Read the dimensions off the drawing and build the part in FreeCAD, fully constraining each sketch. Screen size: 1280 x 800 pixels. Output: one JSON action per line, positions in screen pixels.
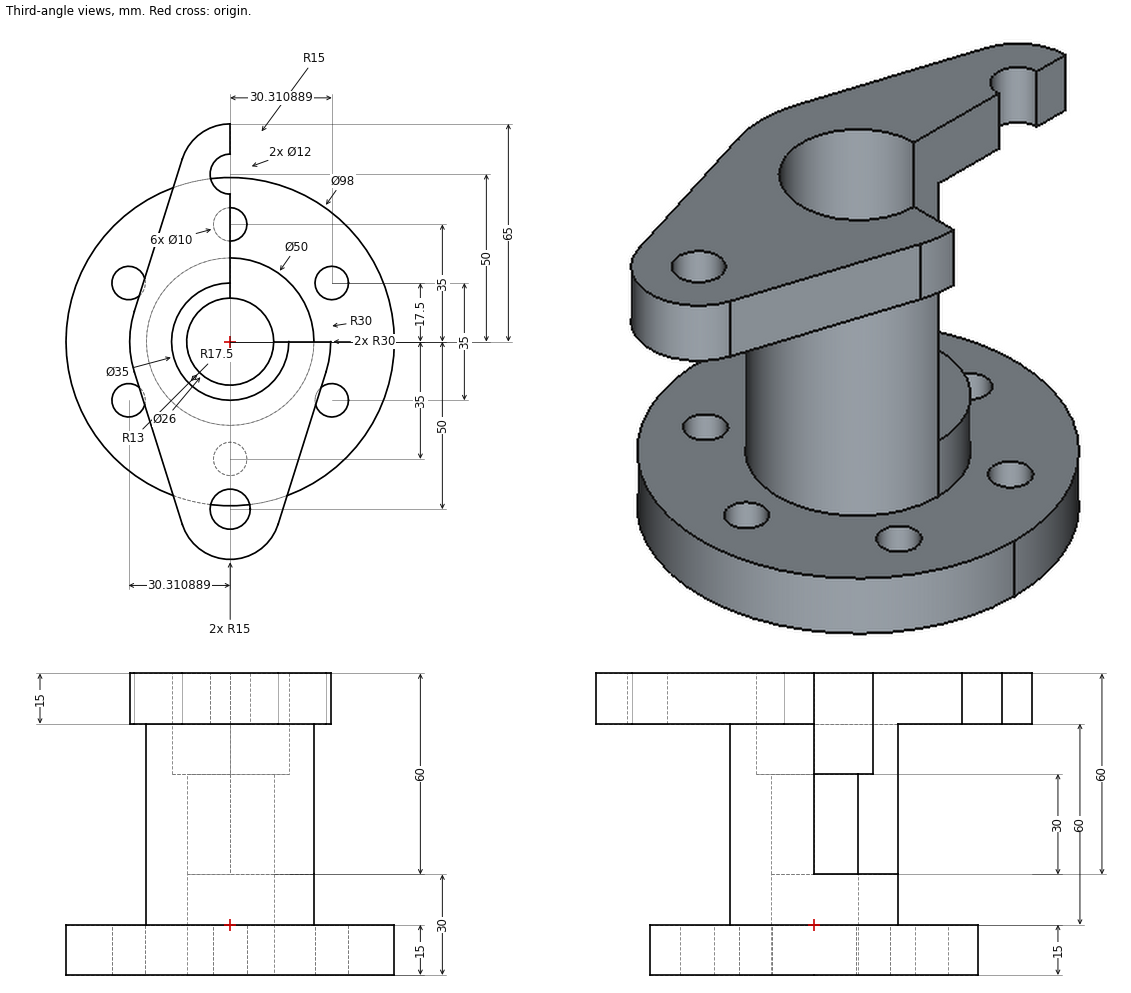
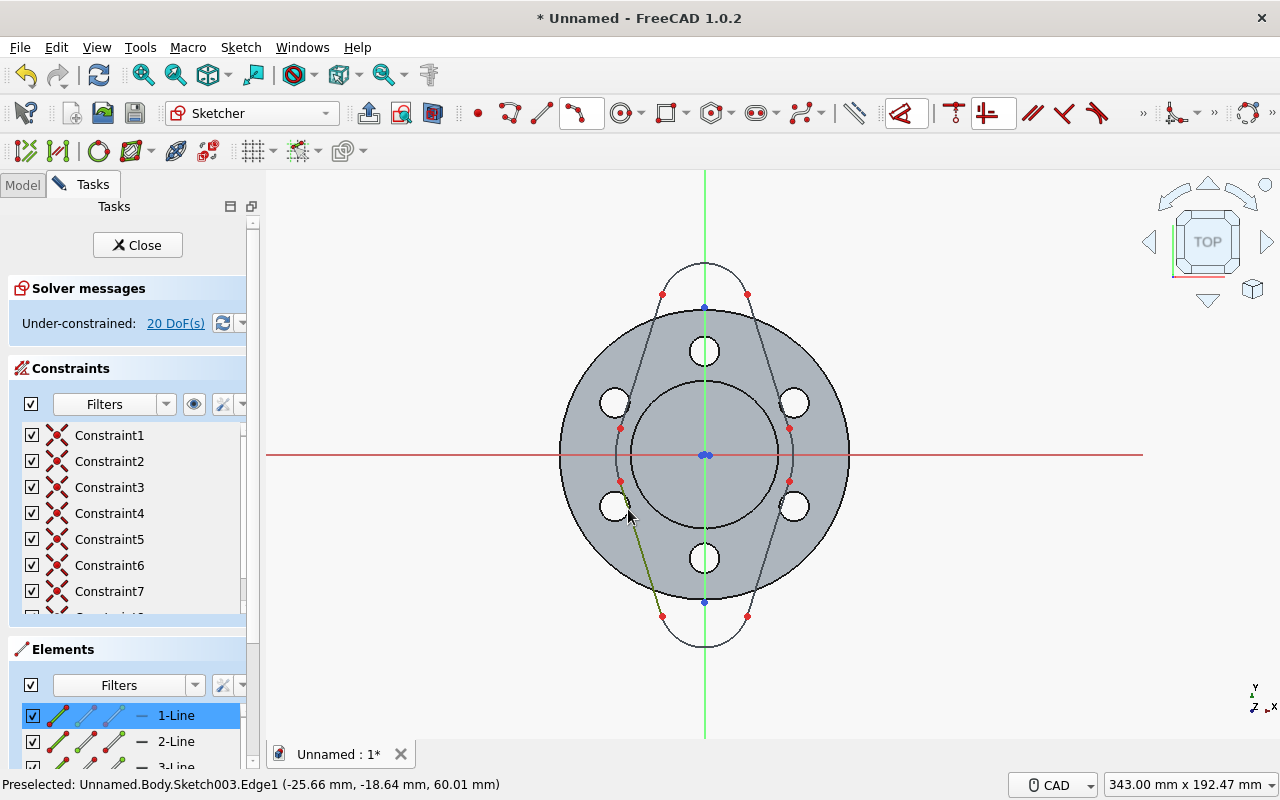
{"action": "left_click", "coordinate": [683, 642]}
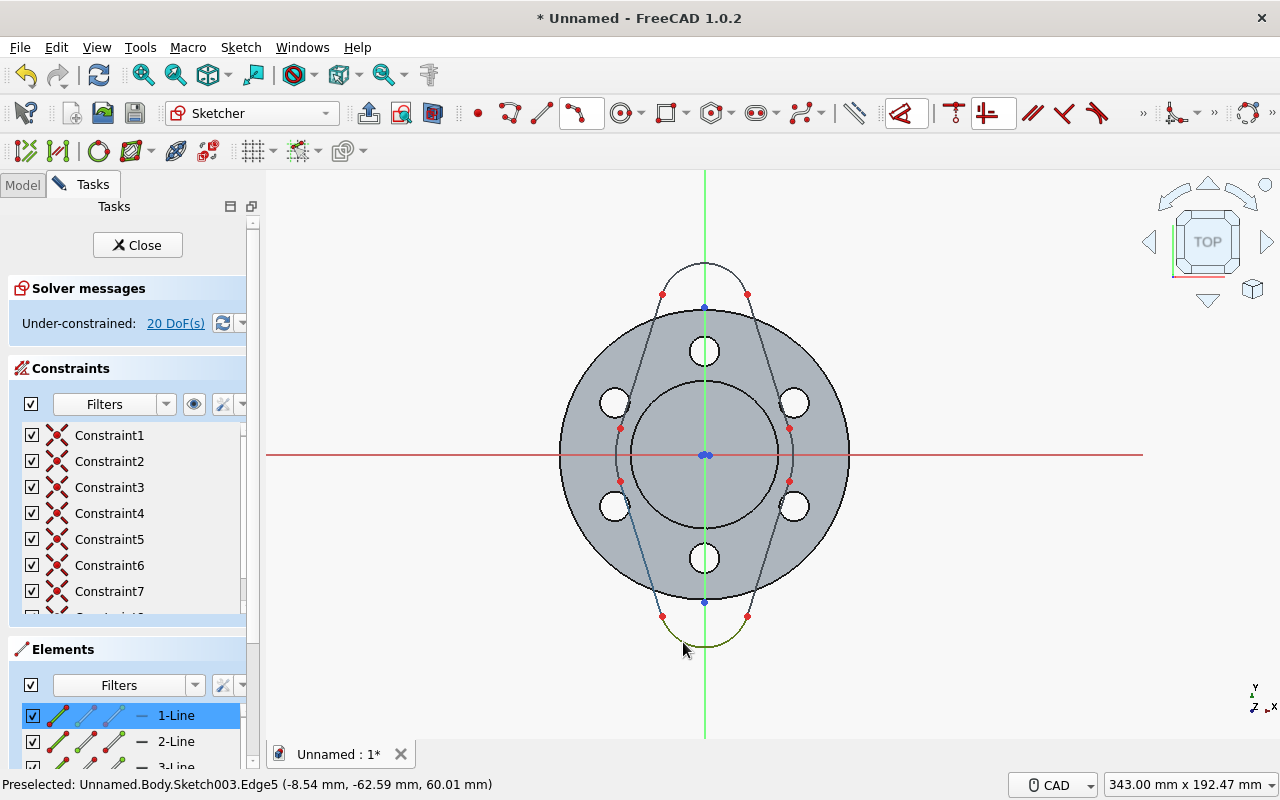
{"action": "left_click", "coordinate": [1098, 114]}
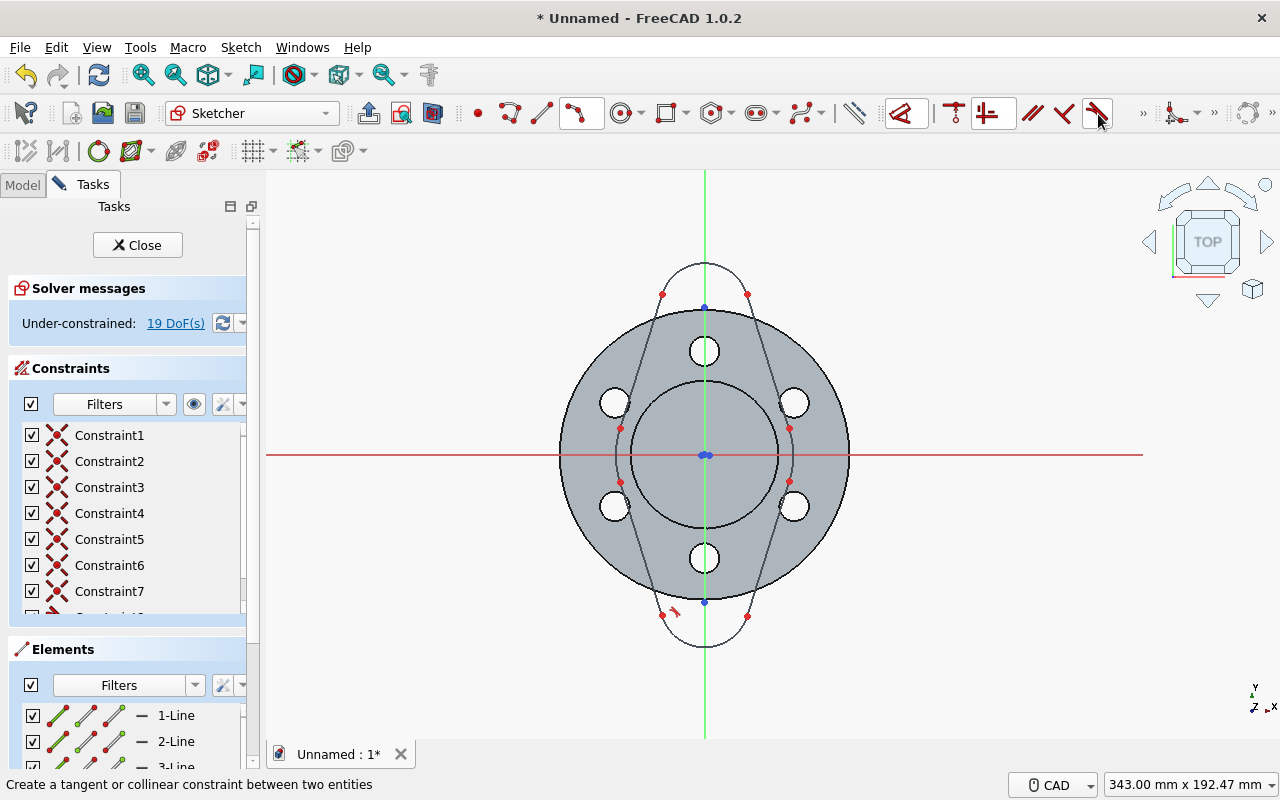
{"action": "left_click", "coordinate": [633, 522]}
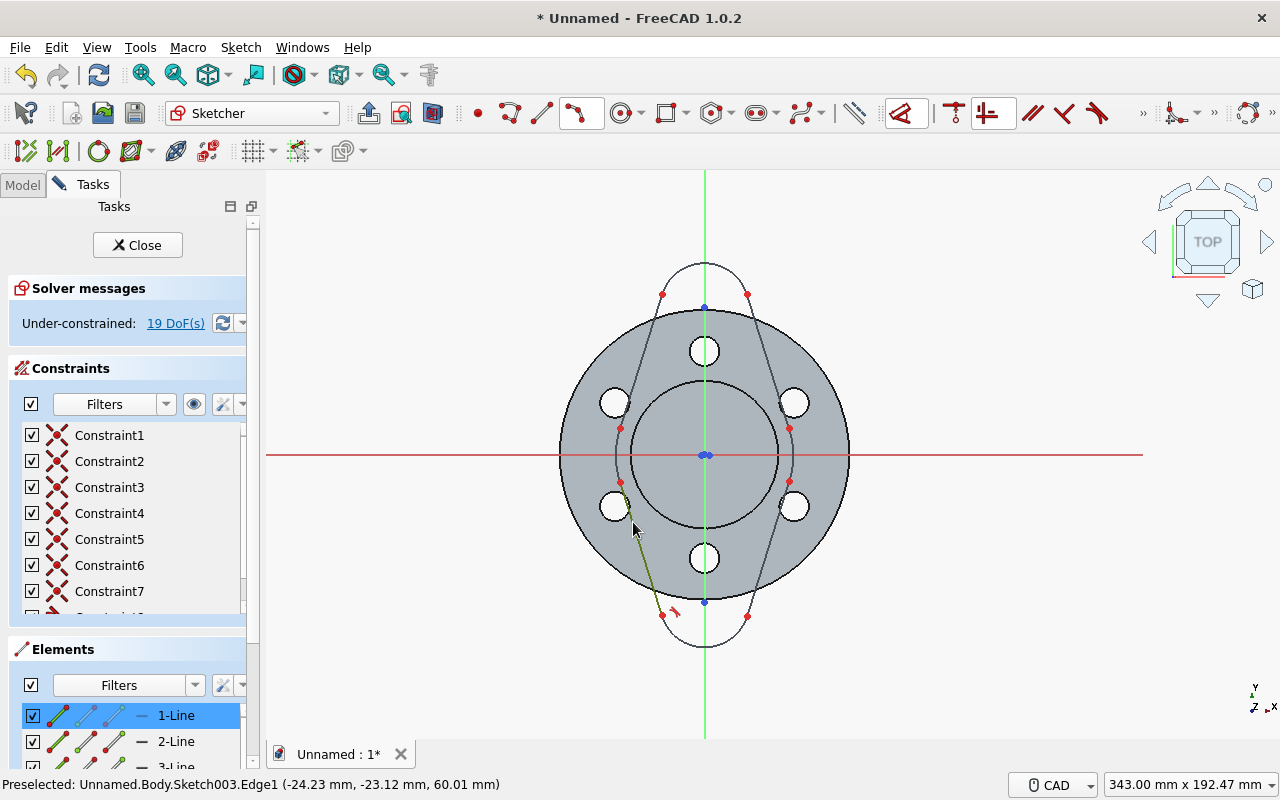
{"action": "scroll", "coordinate": [616, 445], "scroll_direction": "up", "scroll_amount": 2}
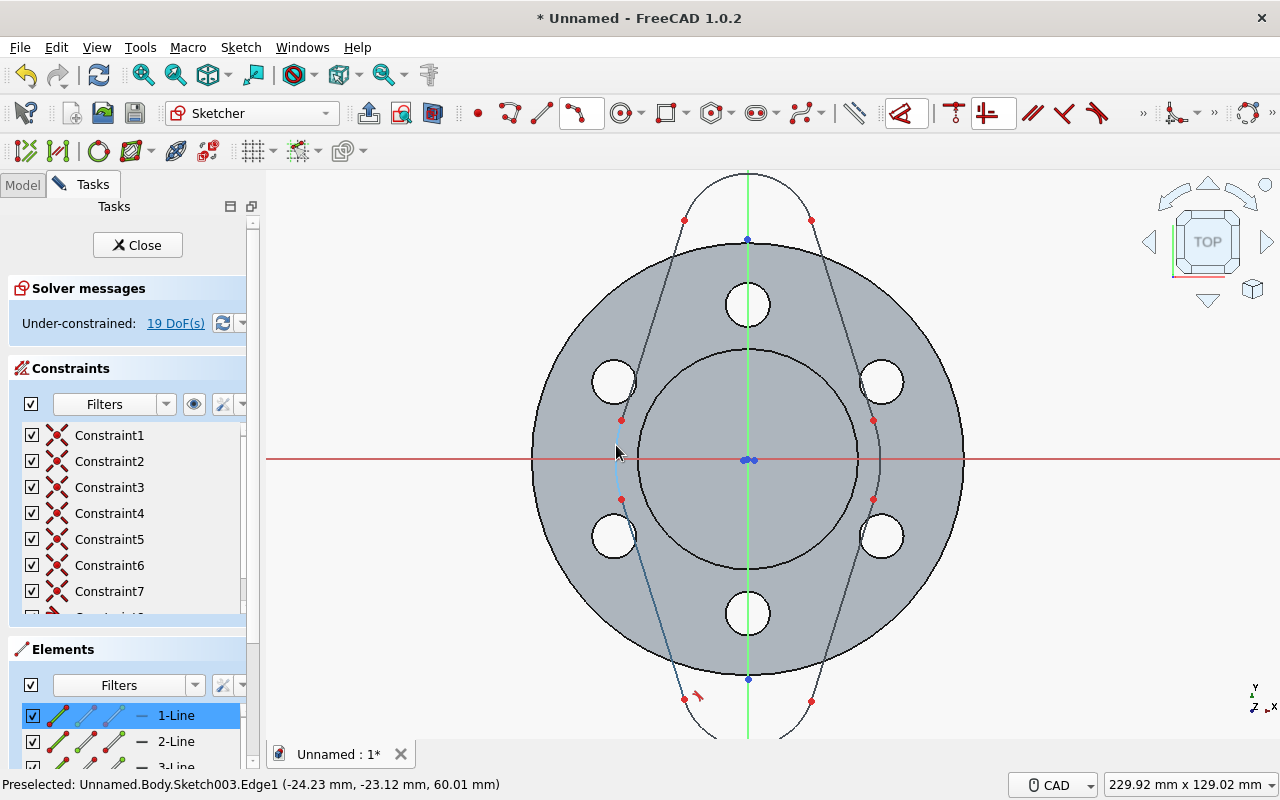
{"action": "left_click", "coordinate": [617, 444]}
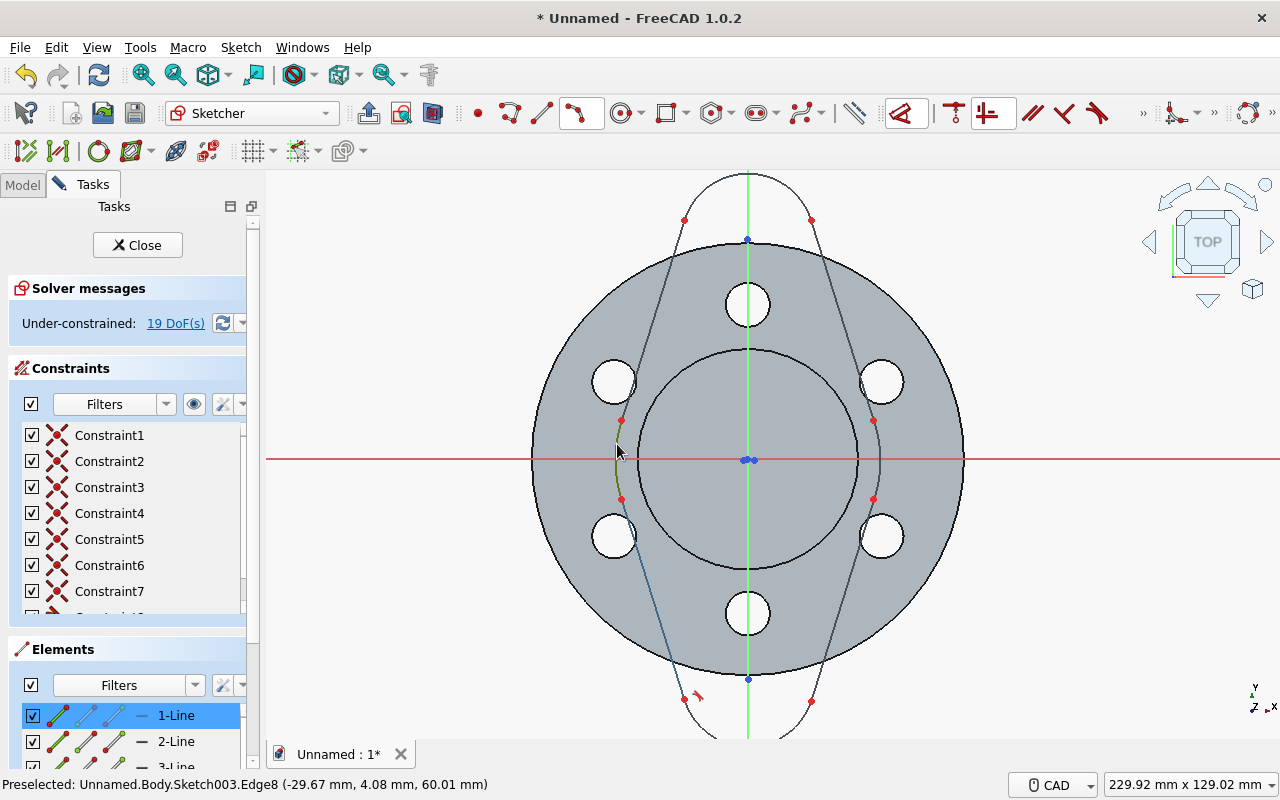
{"action": "left_click", "coordinate": [1098, 114]}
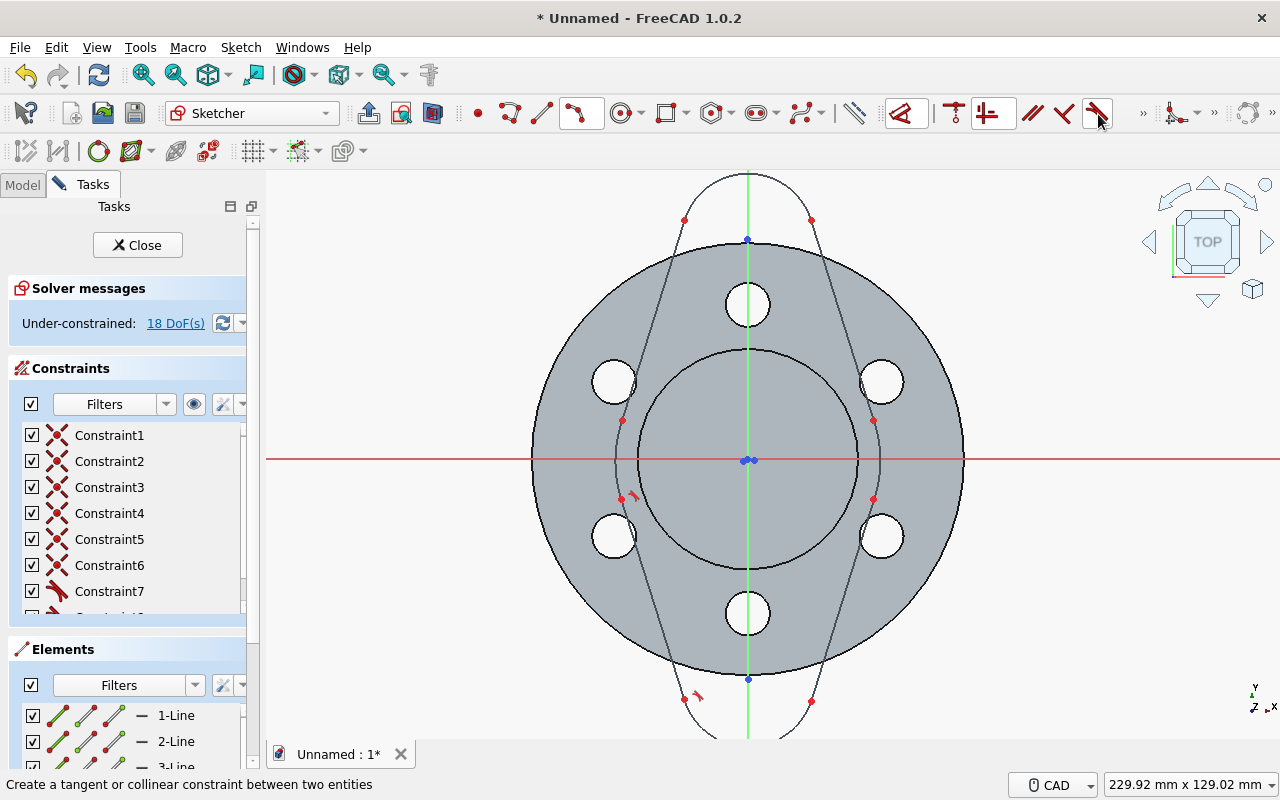
{"action": "left_click", "coordinate": [830, 641]}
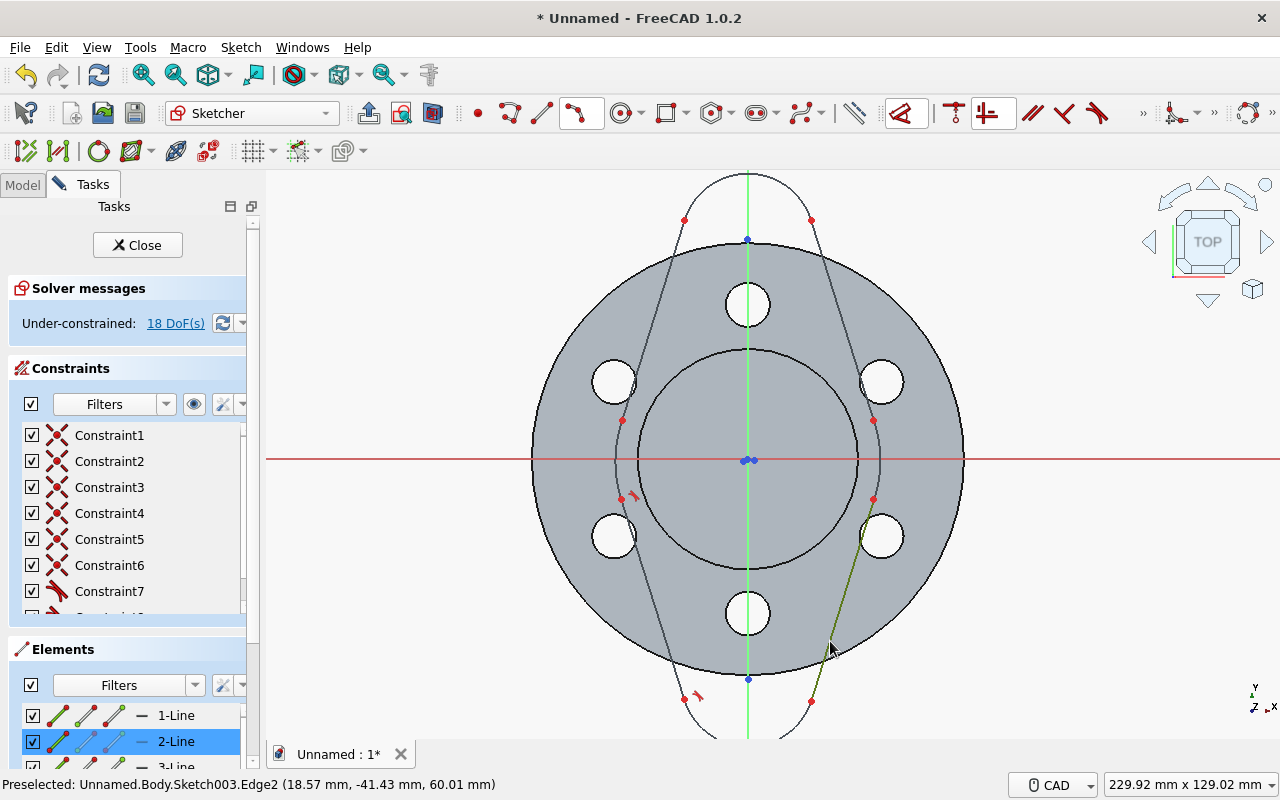
{"action": "scroll", "coordinate": [616, 445], "scroll_direction": "down", "scroll_amount": 2}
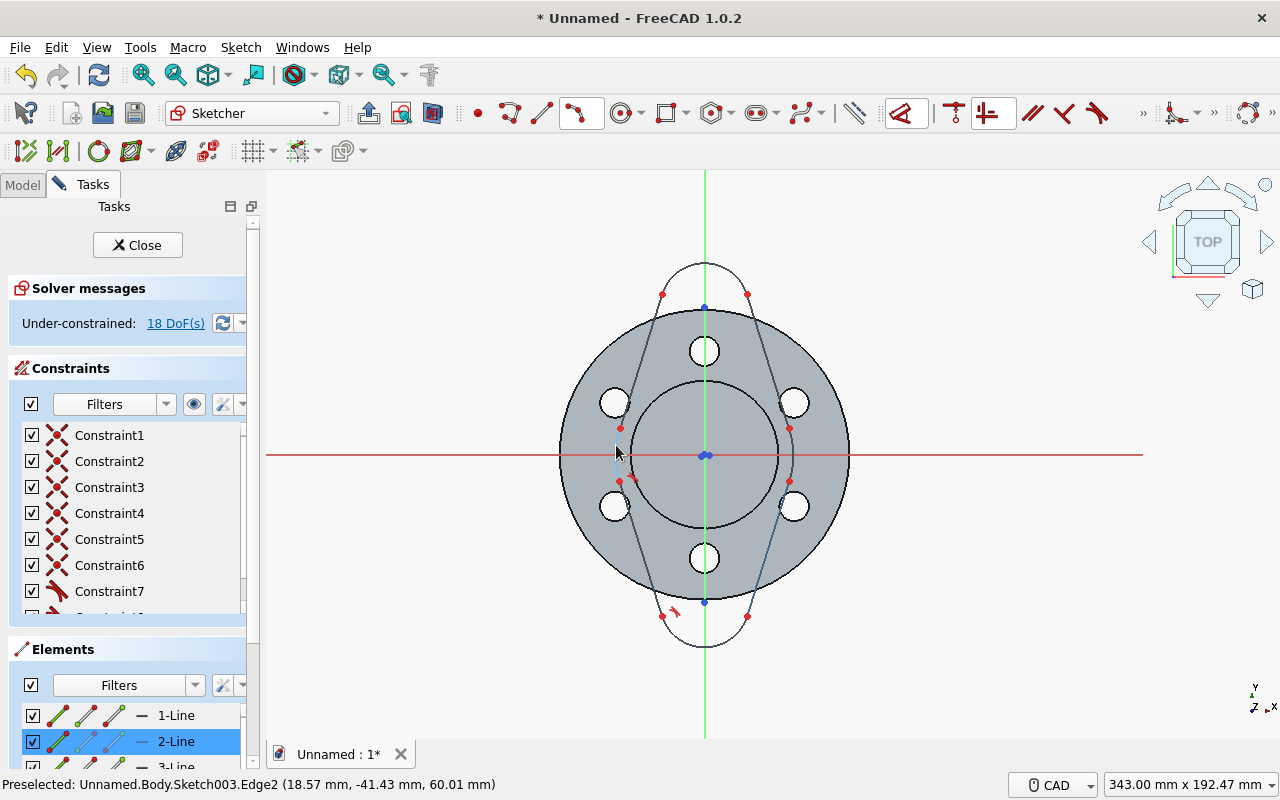
{"action": "left_click", "coordinate": [683, 642]}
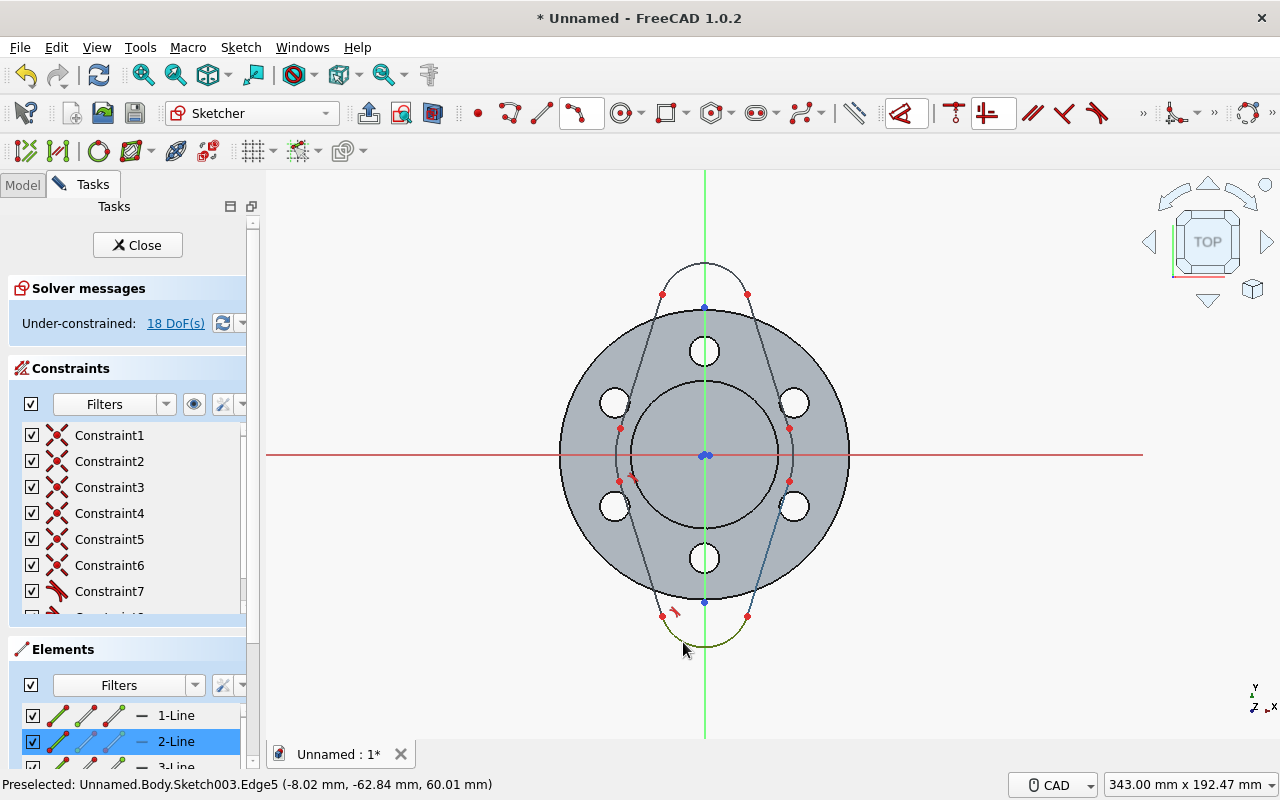
{"action": "left_click", "coordinate": [1098, 114]}